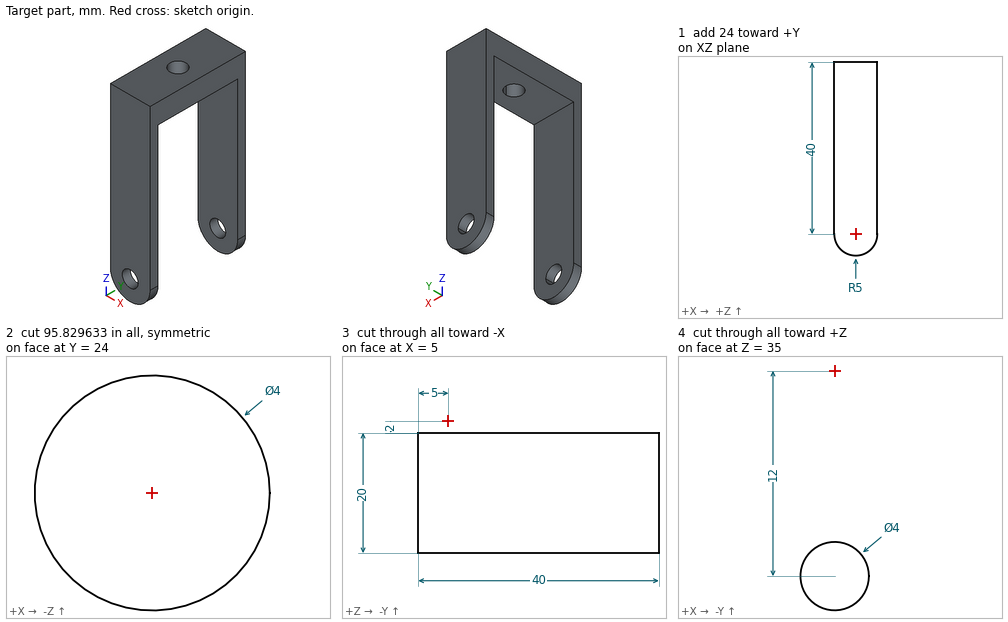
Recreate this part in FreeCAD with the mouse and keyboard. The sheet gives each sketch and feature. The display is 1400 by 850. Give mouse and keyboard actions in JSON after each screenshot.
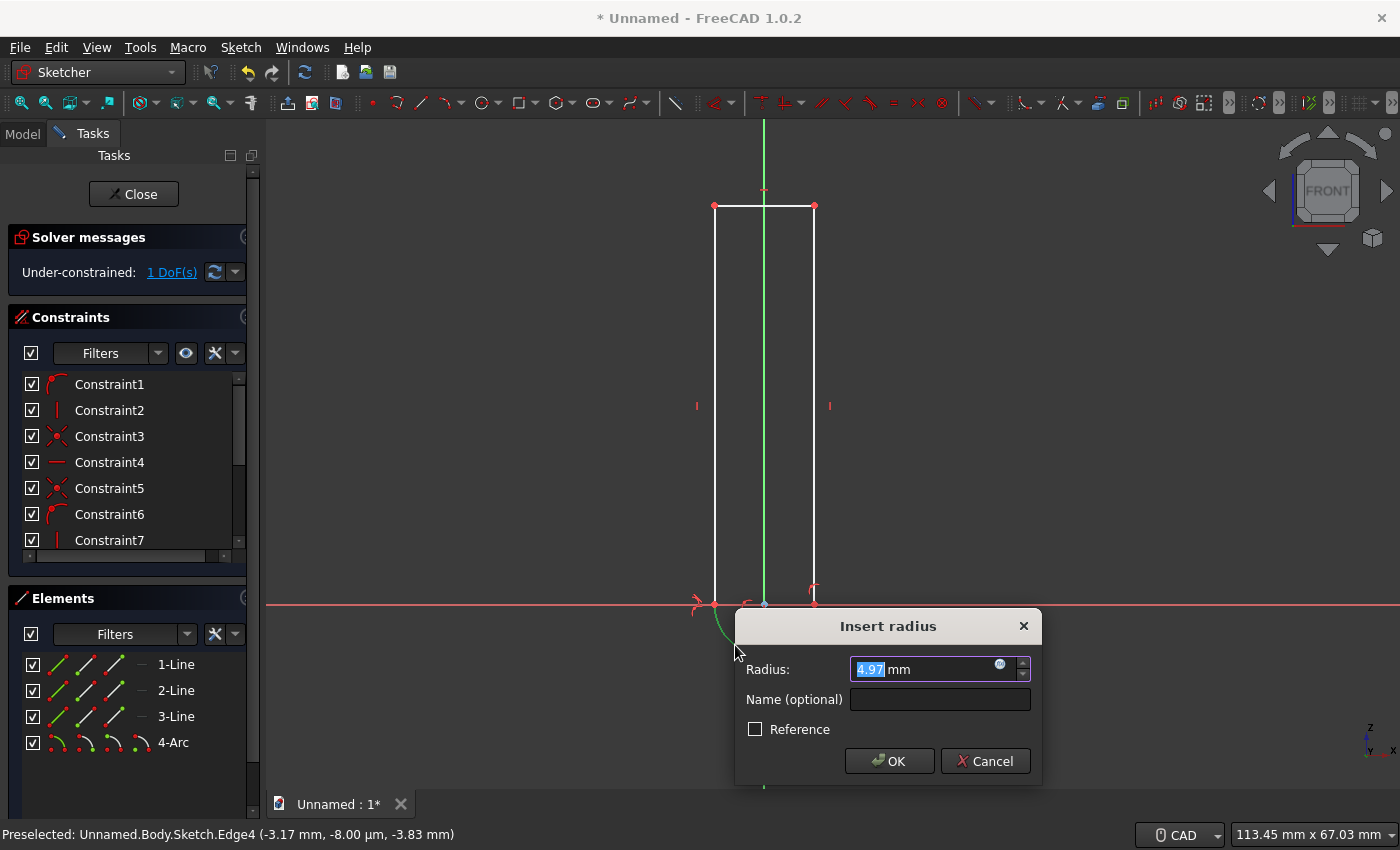
{"action": "type", "text": "5"}
{"action": "key", "text": "Return"}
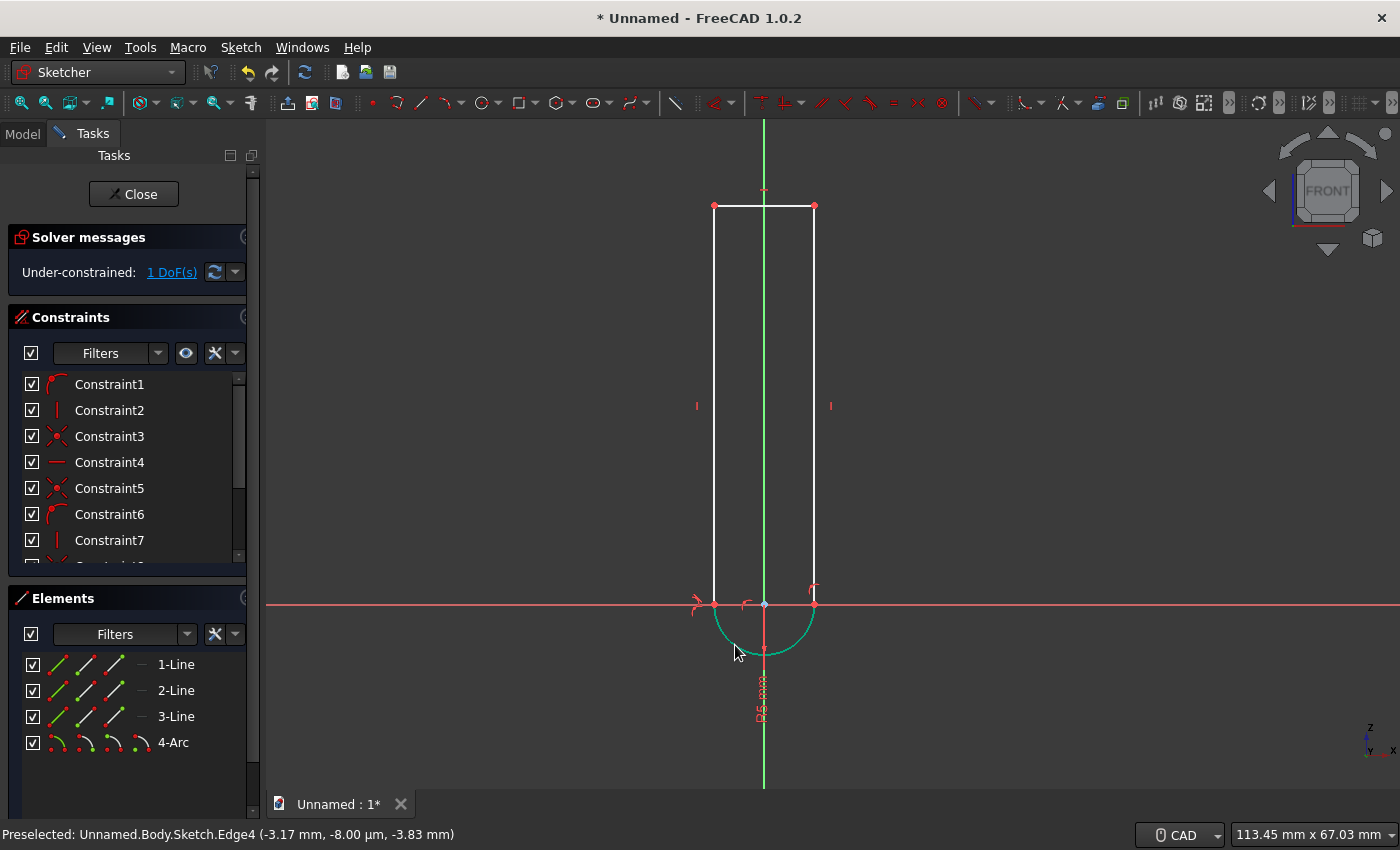
{"action": "left_click", "coordinate": [714, 485]}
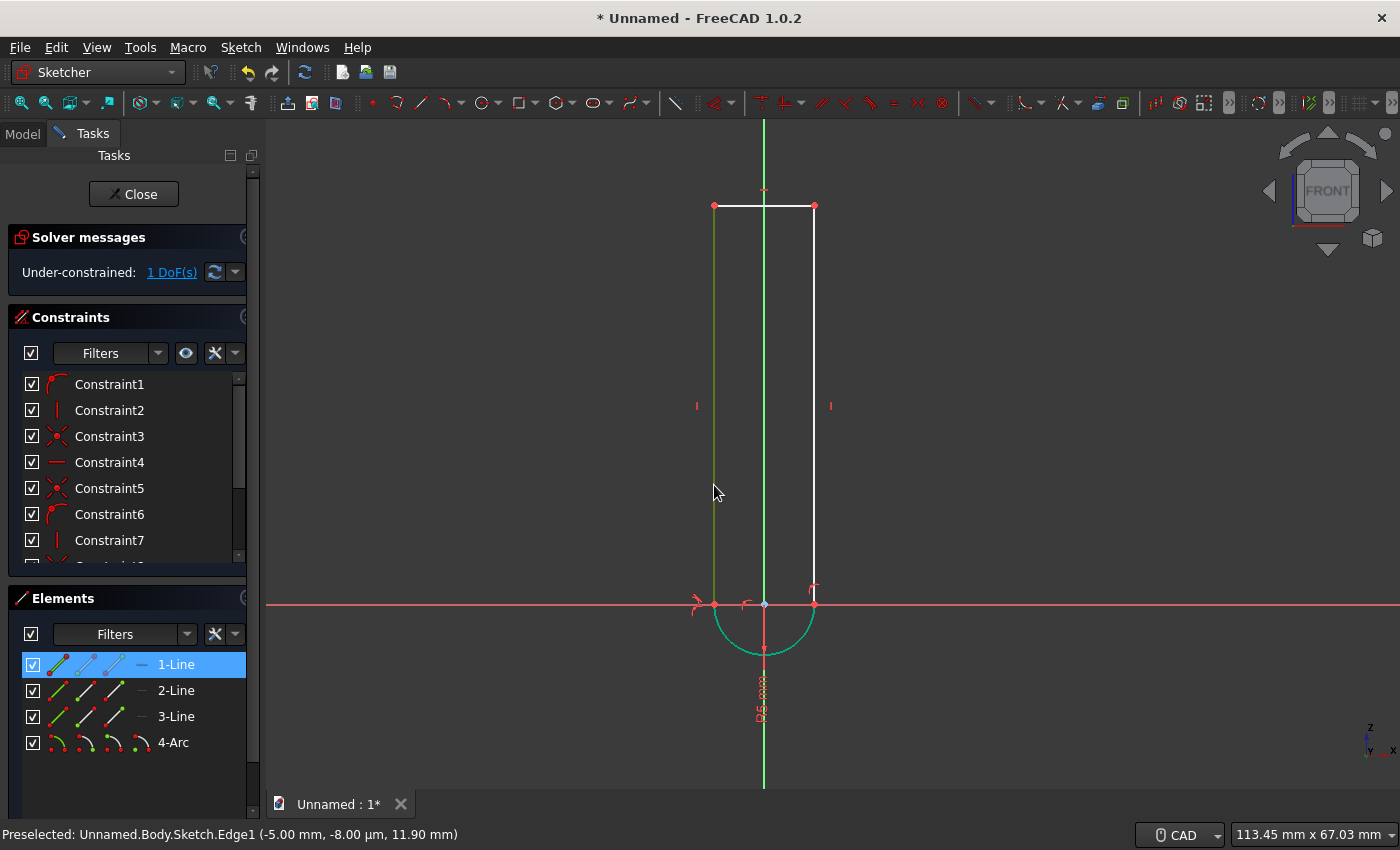
{"action": "key", "text": "i"}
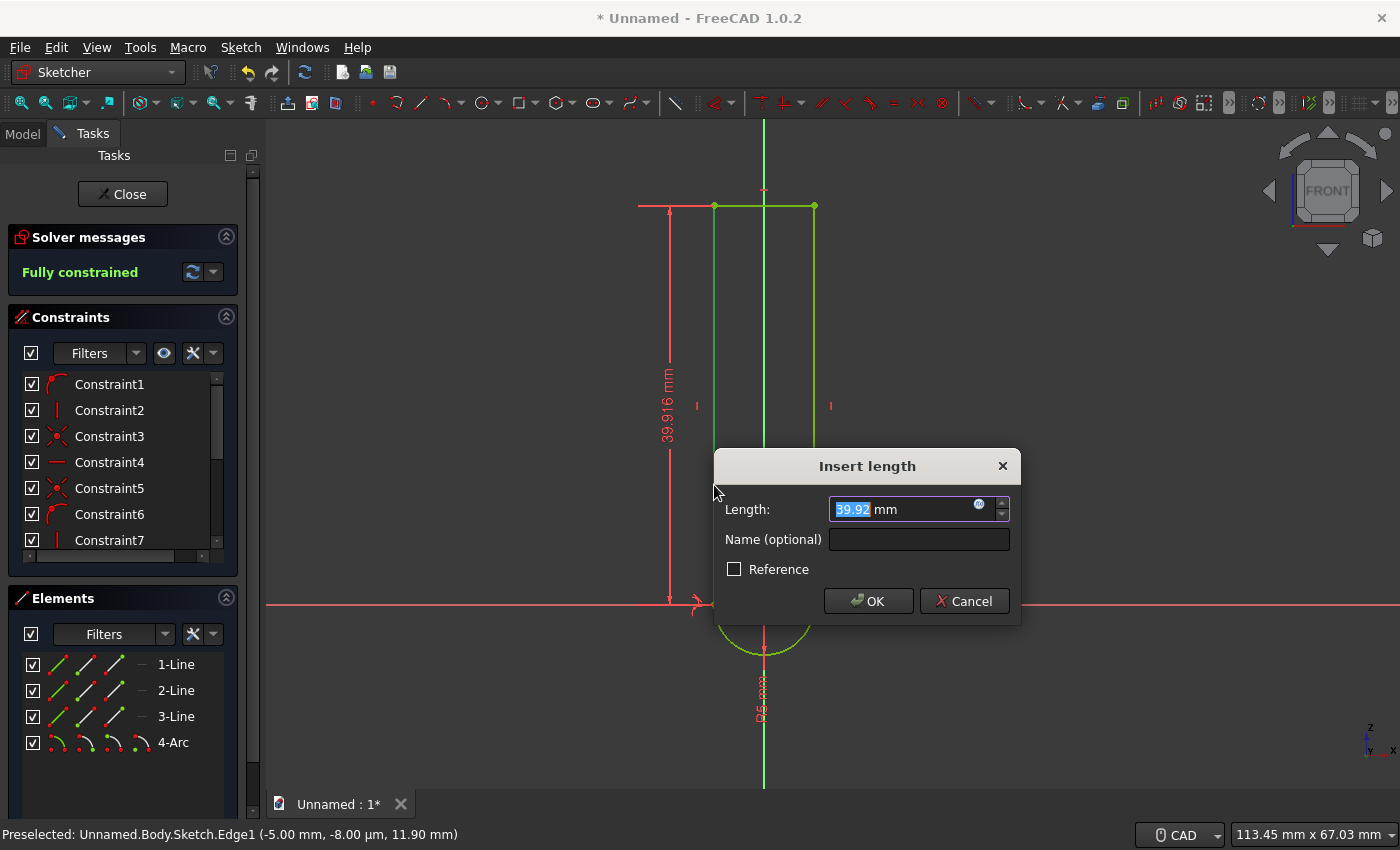
{"action": "type", "text": "40"}
{"action": "key", "text": "Return"}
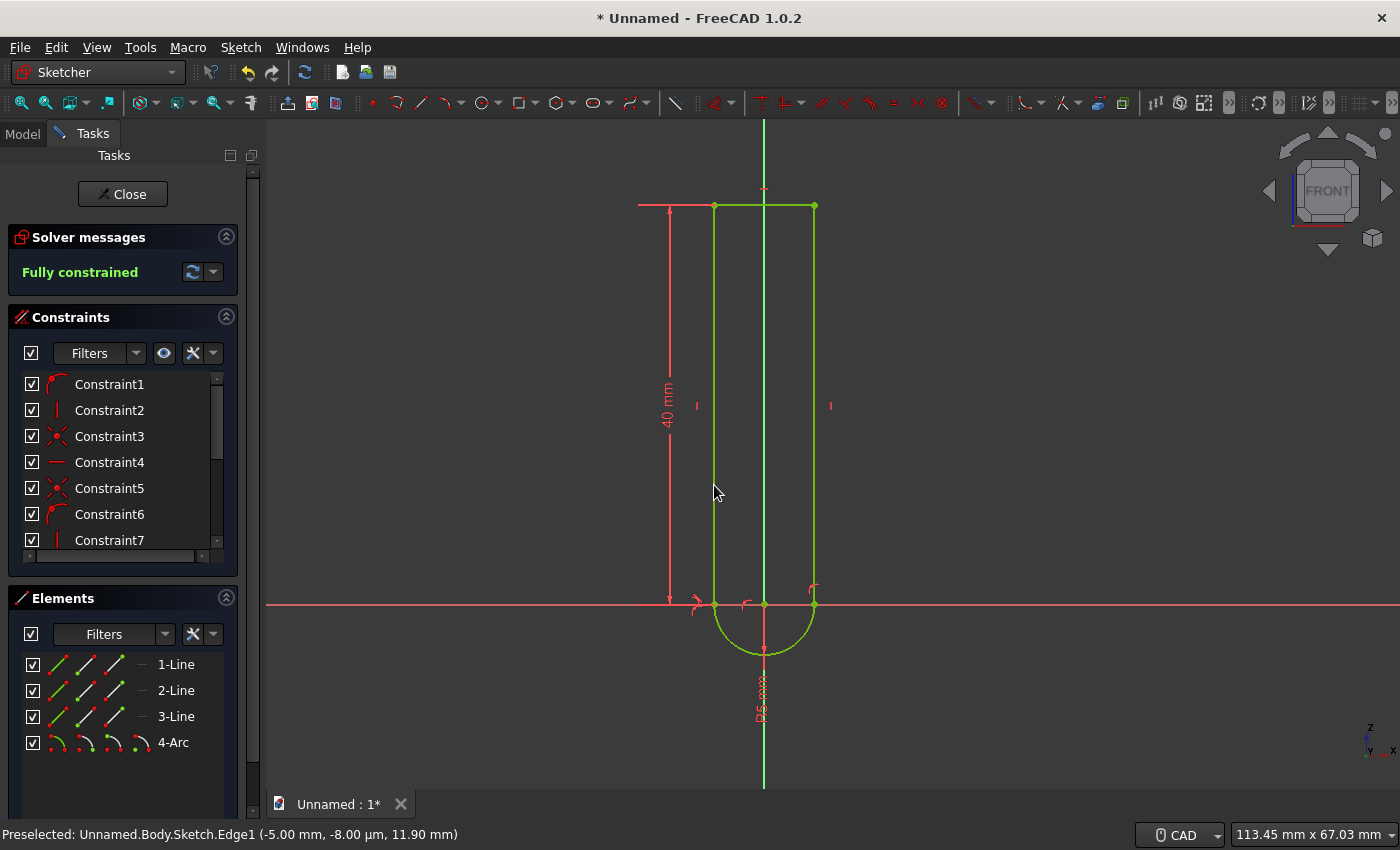
{"action": "left_click", "coordinate": [123, 194]}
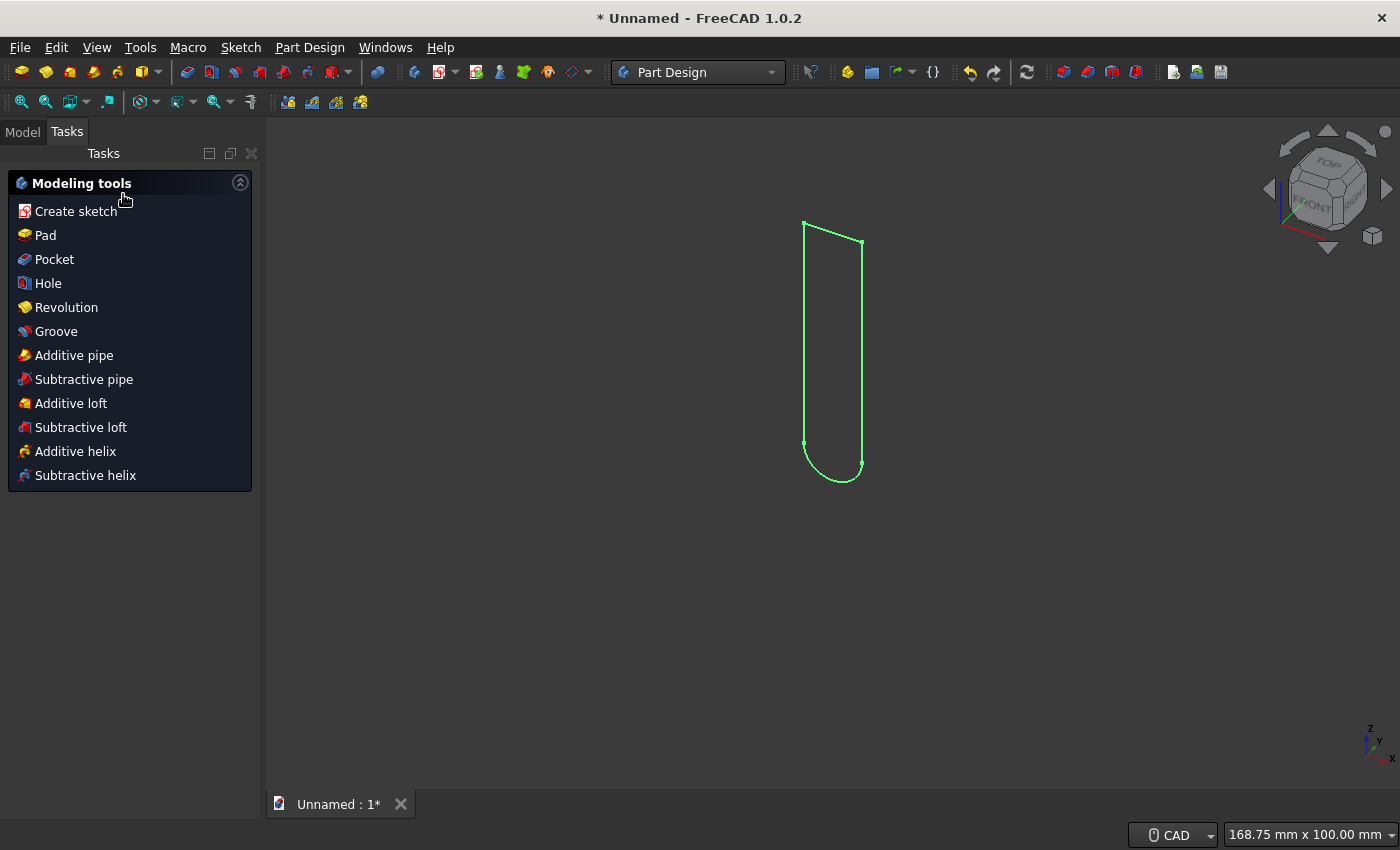
{"action": "left_click", "coordinate": [22, 72]}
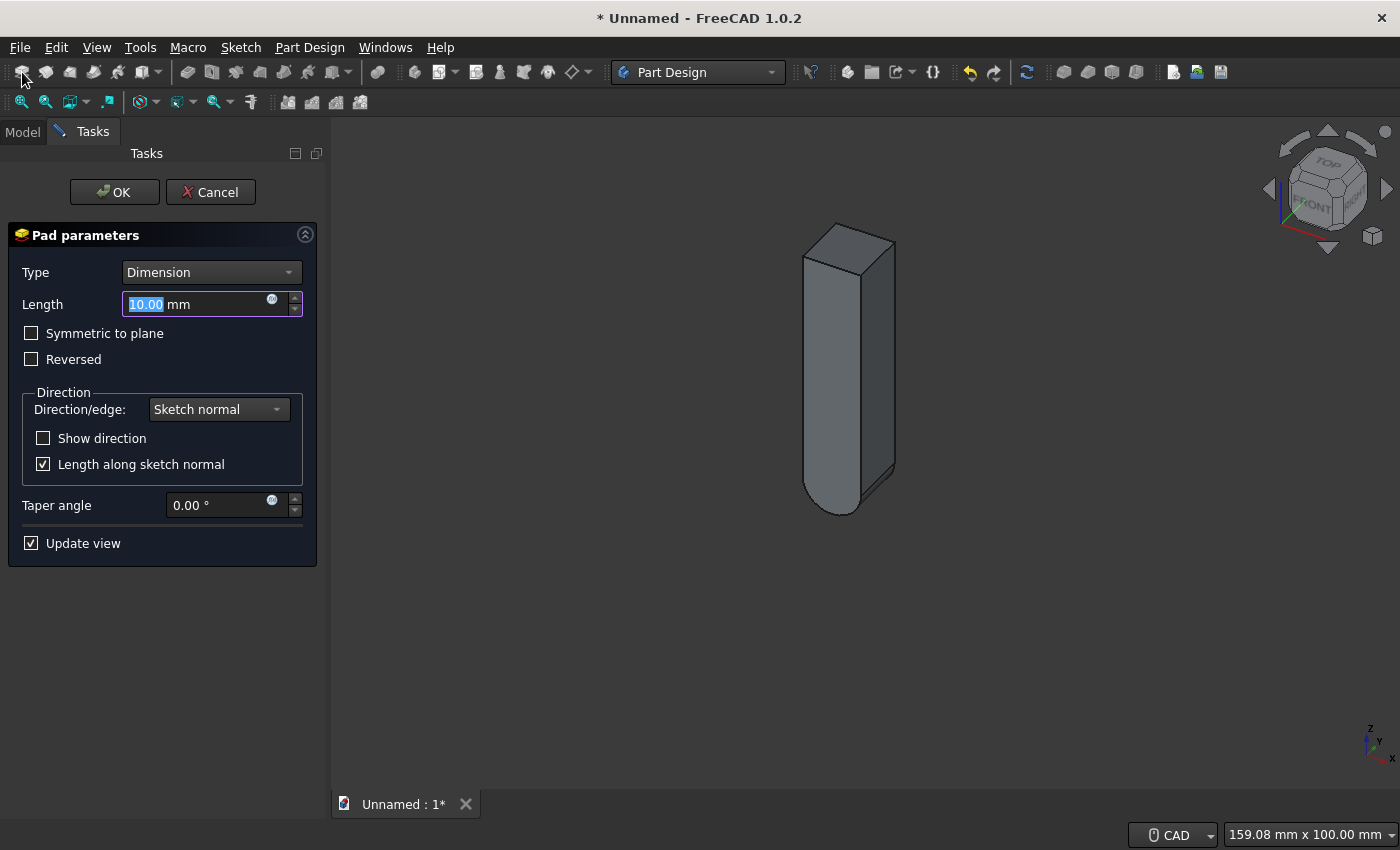
{"action": "type", "text": "24"}
{"action": "key", "text": "Tab"}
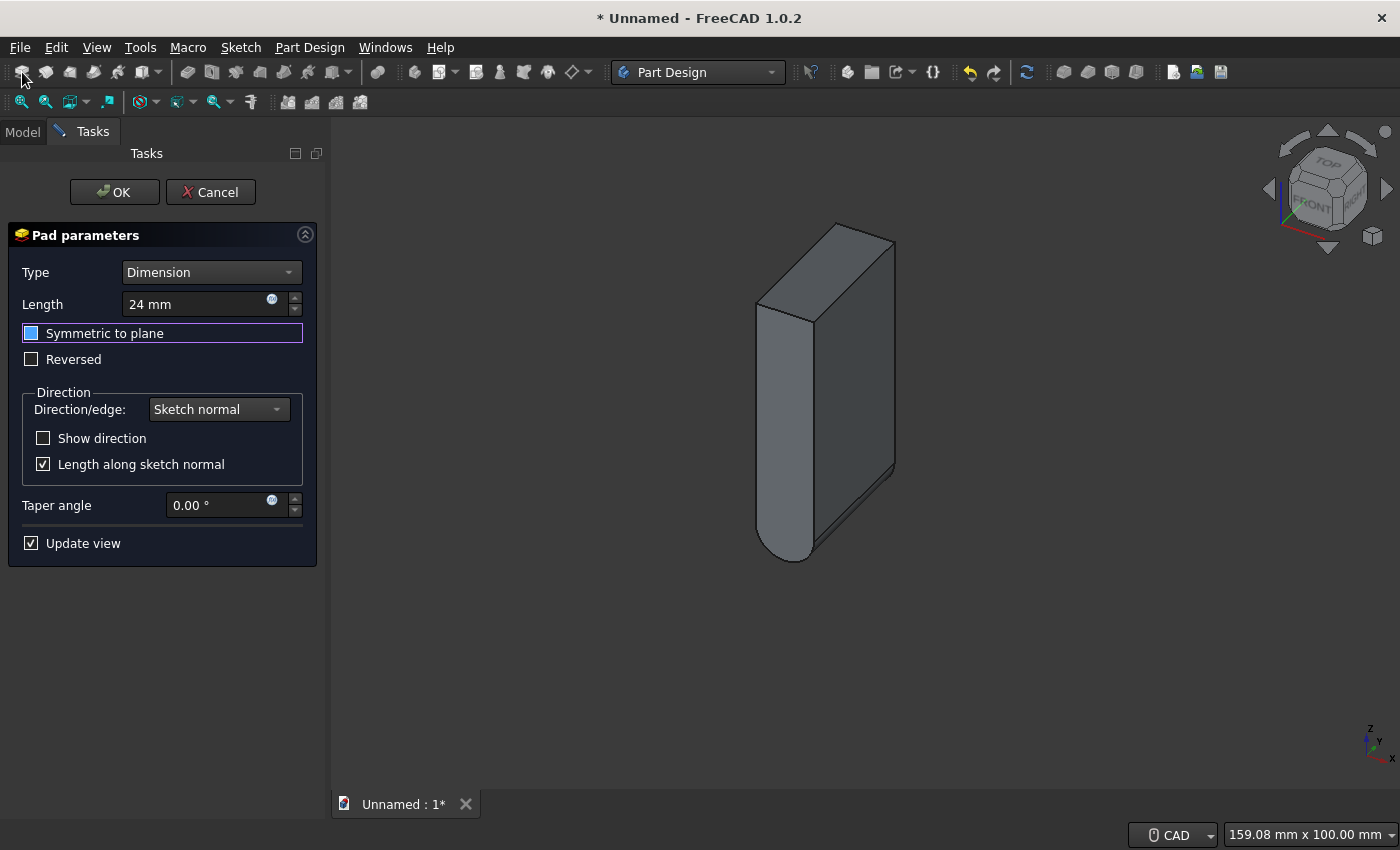
{"action": "left_click", "coordinate": [30, 359]}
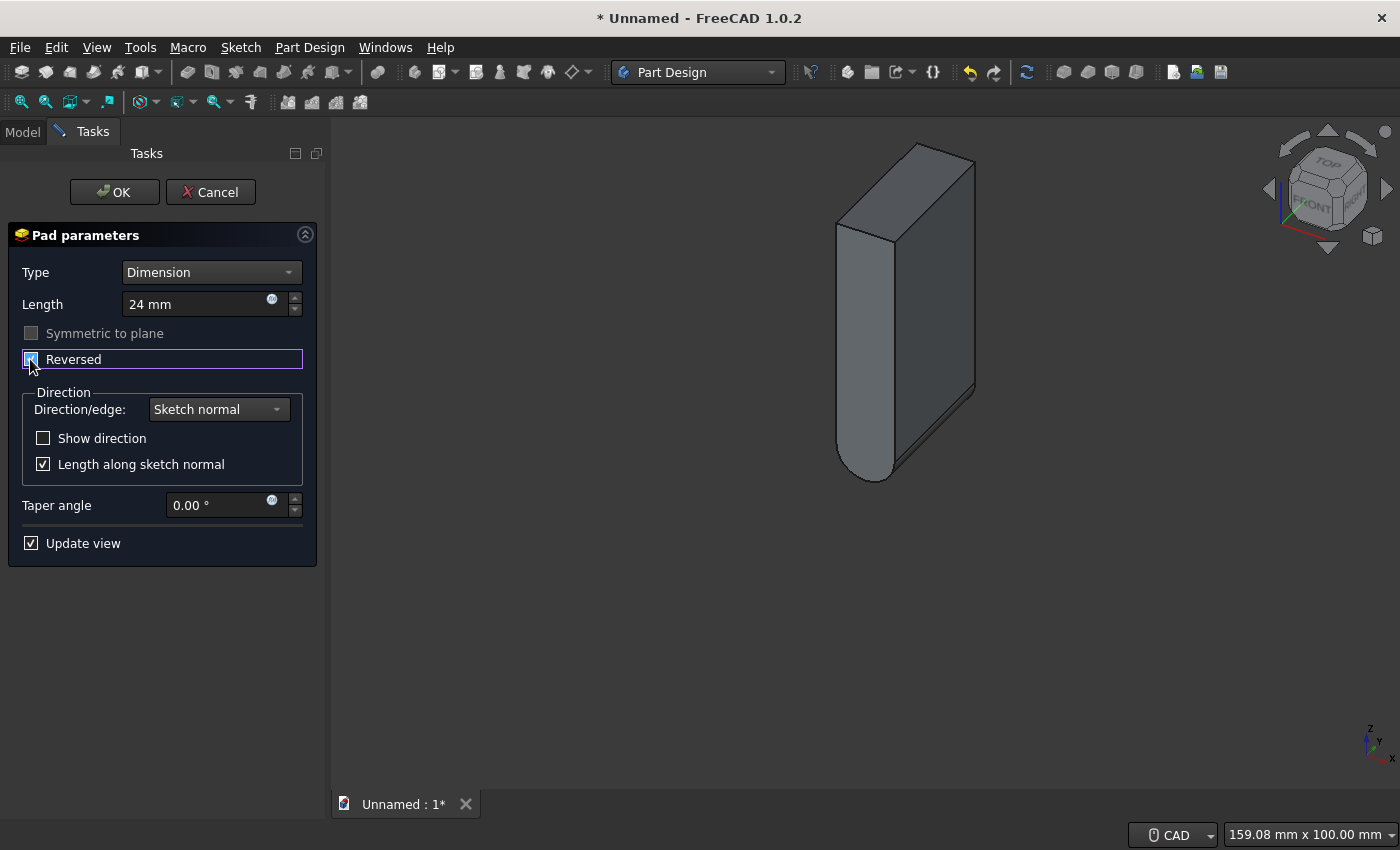
{"action": "left_click", "coordinate": [115, 192]}